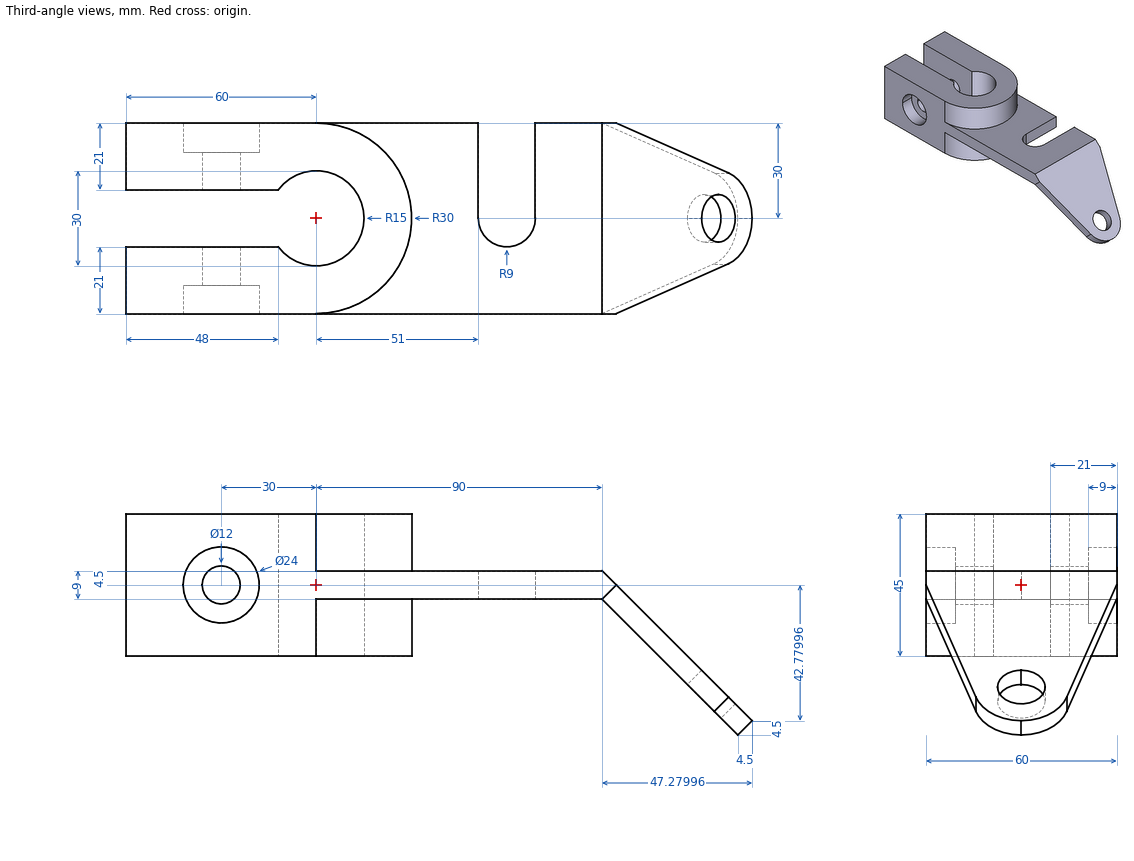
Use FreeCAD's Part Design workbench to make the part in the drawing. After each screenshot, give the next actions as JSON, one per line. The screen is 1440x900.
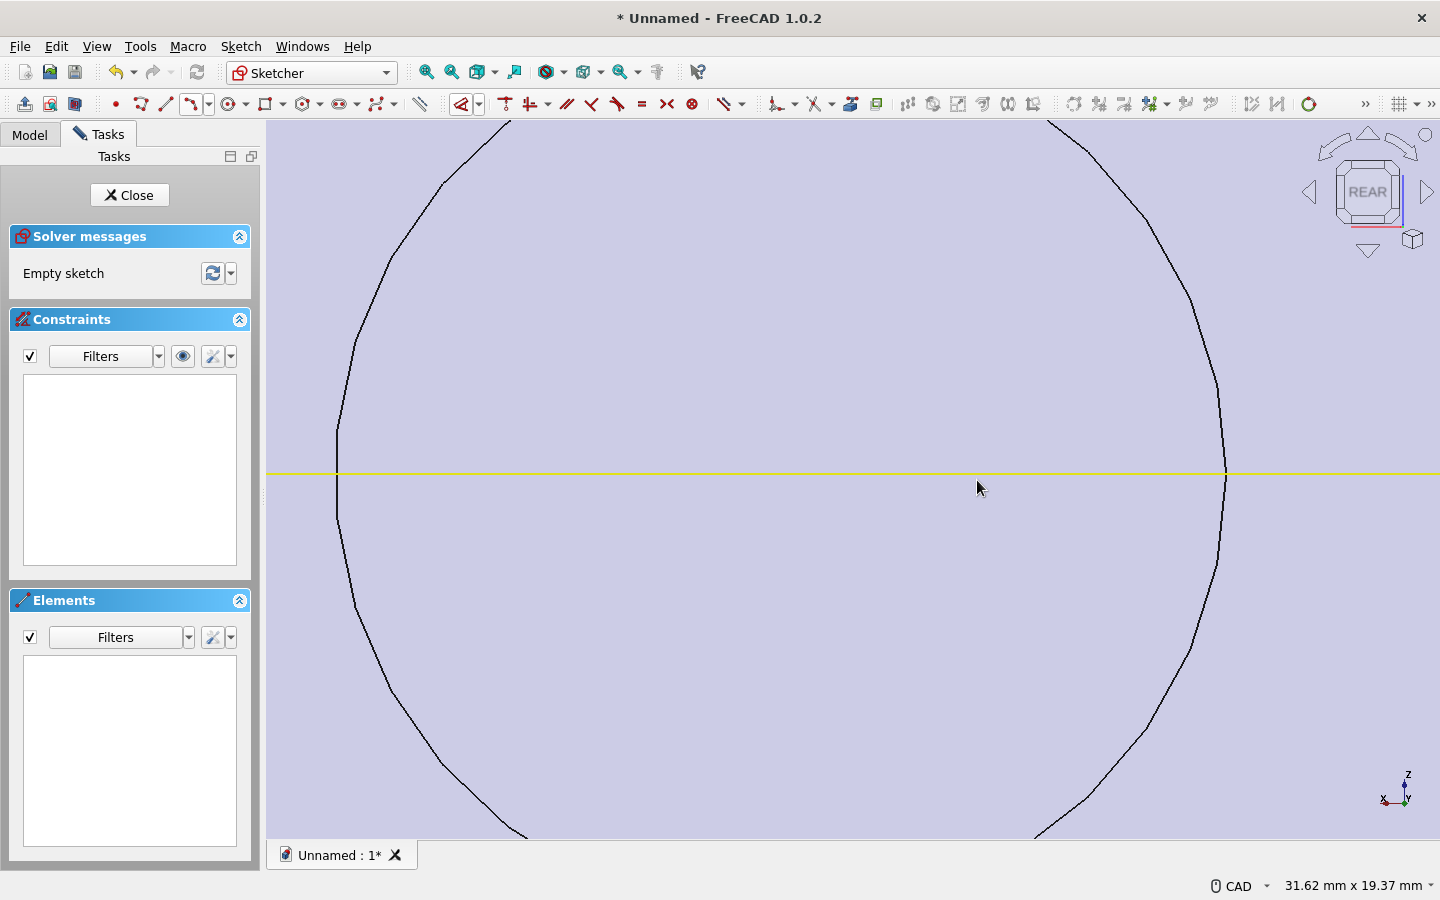
{"action": "key", "text": "g c"}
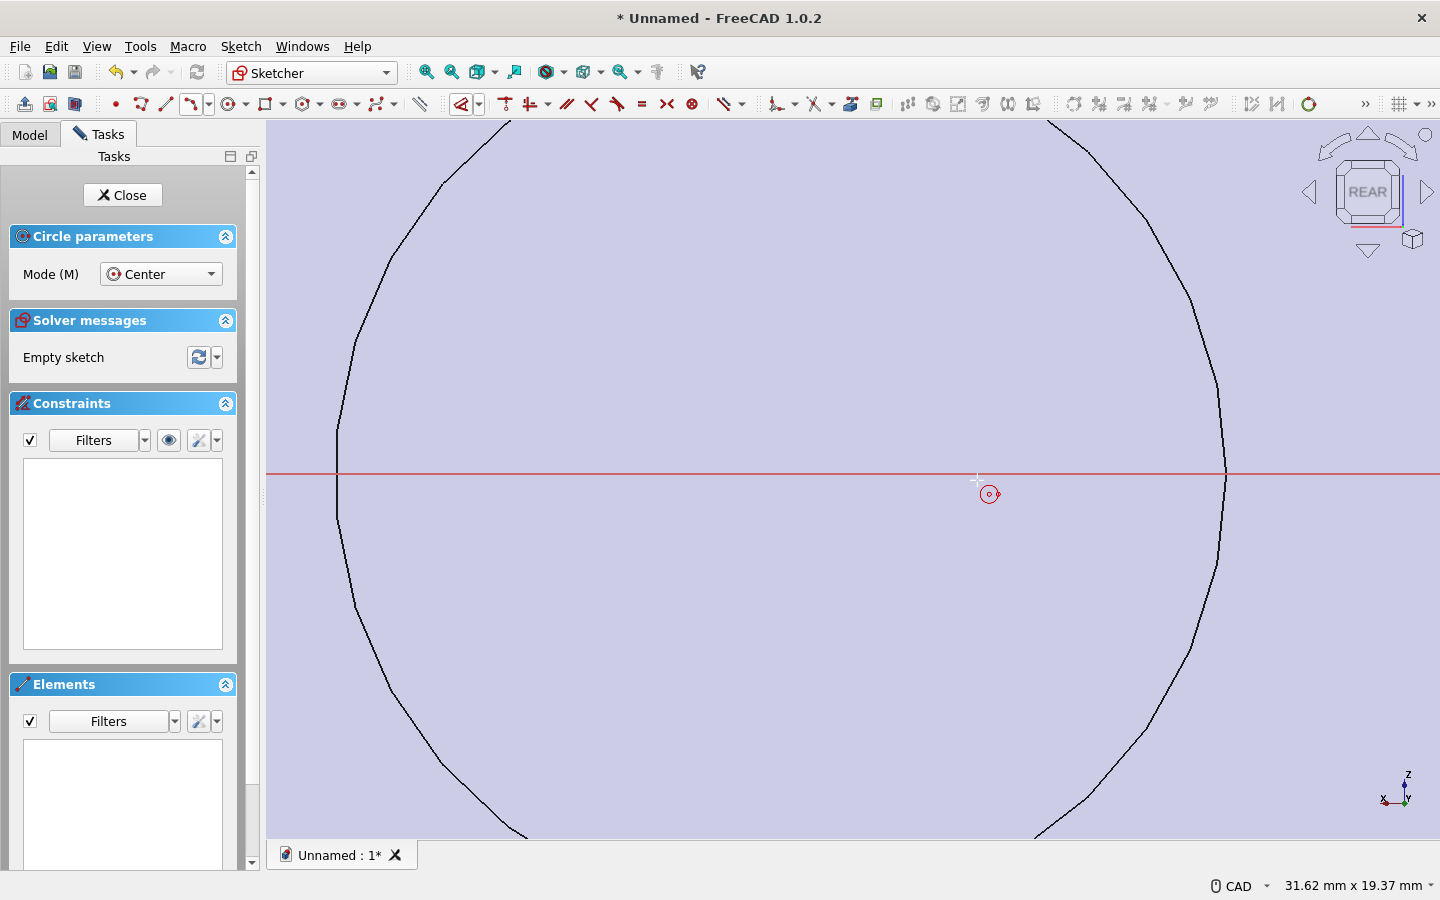
{"action": "left_click", "coordinate": [781, 474]}
{"action": "left_click", "coordinate": [938, 317]}
{"action": "key", "text": "Escape"}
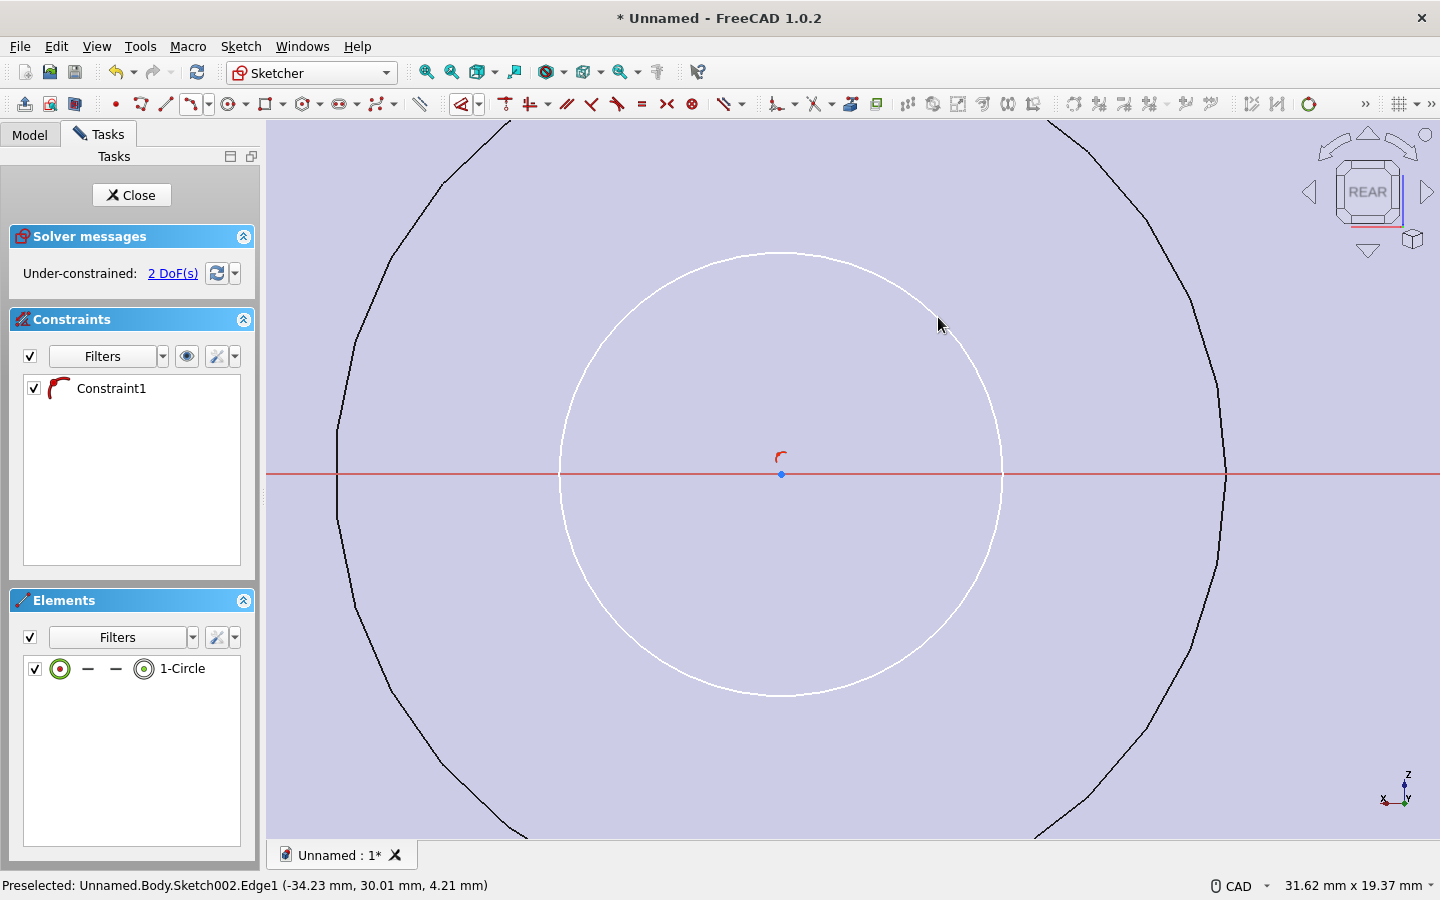
{"action": "left_click", "coordinate": [937, 317]}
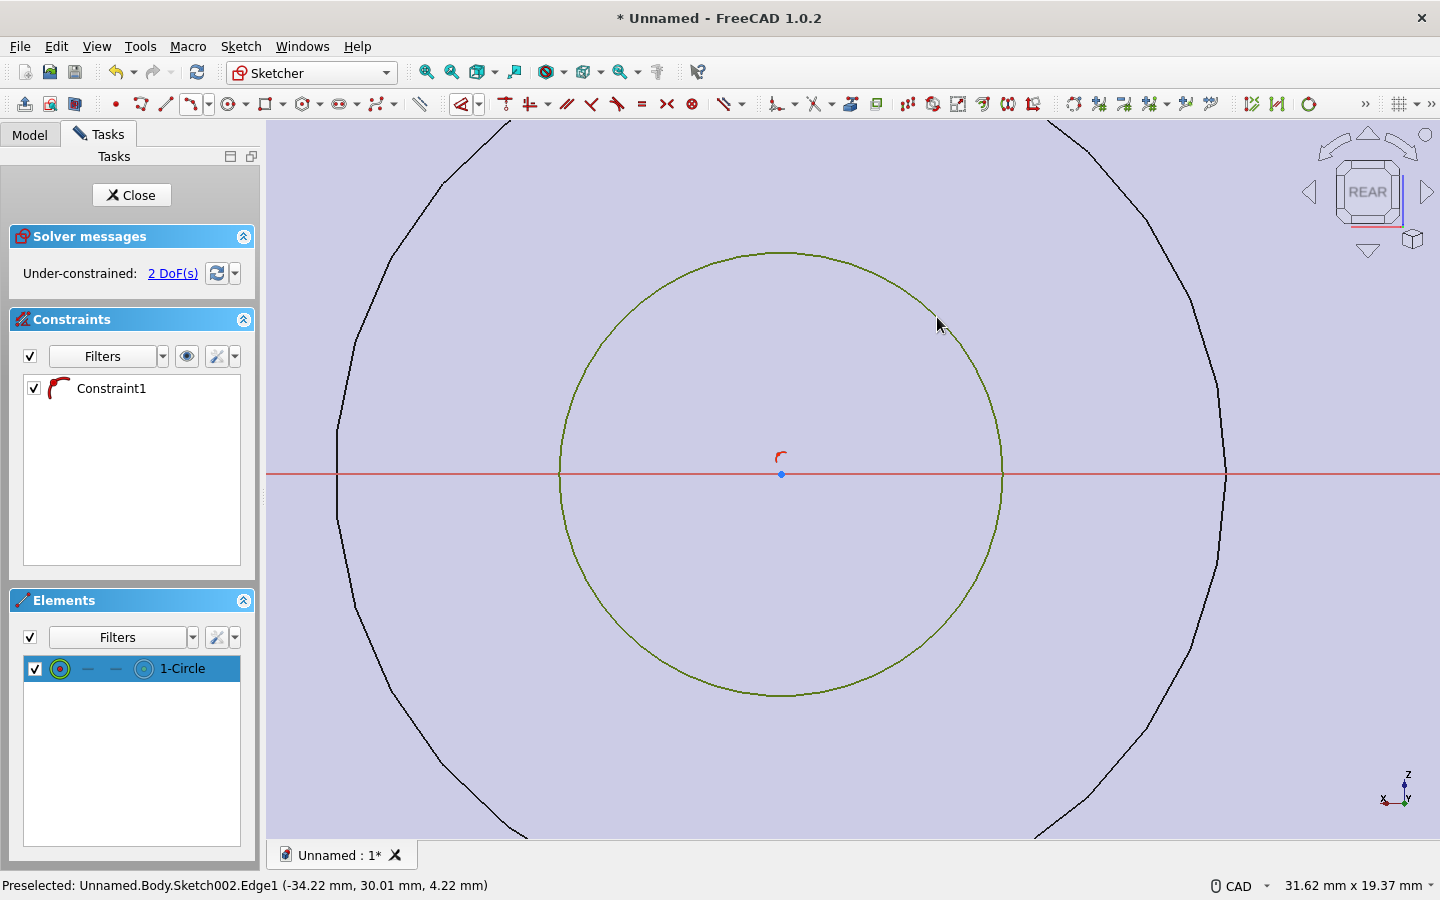
{"action": "left_click", "coordinate": [478, 104]}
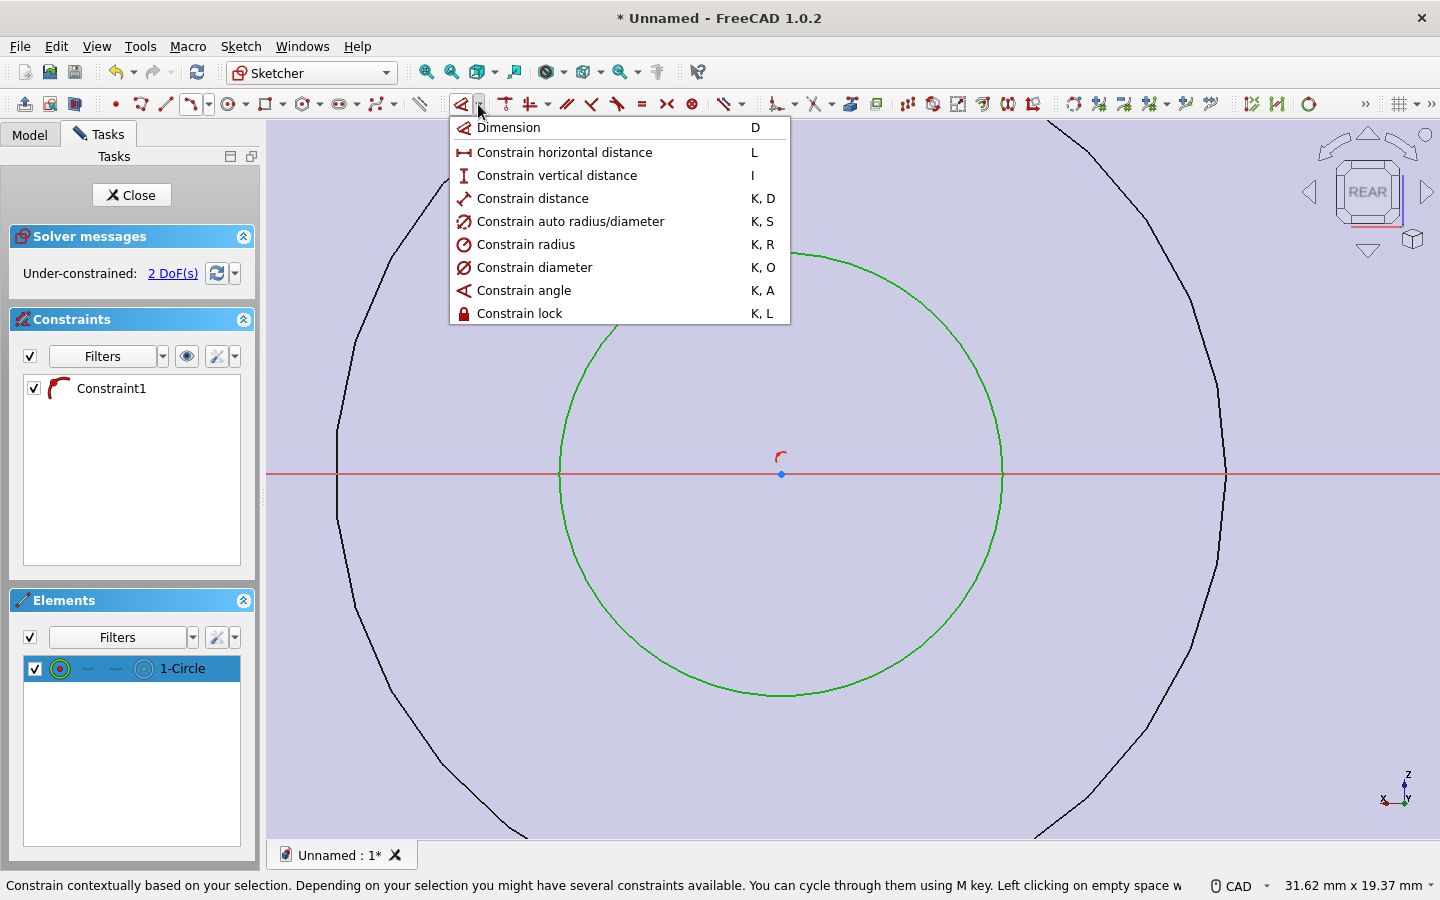
{"action": "left_click", "coordinate": [620, 268]}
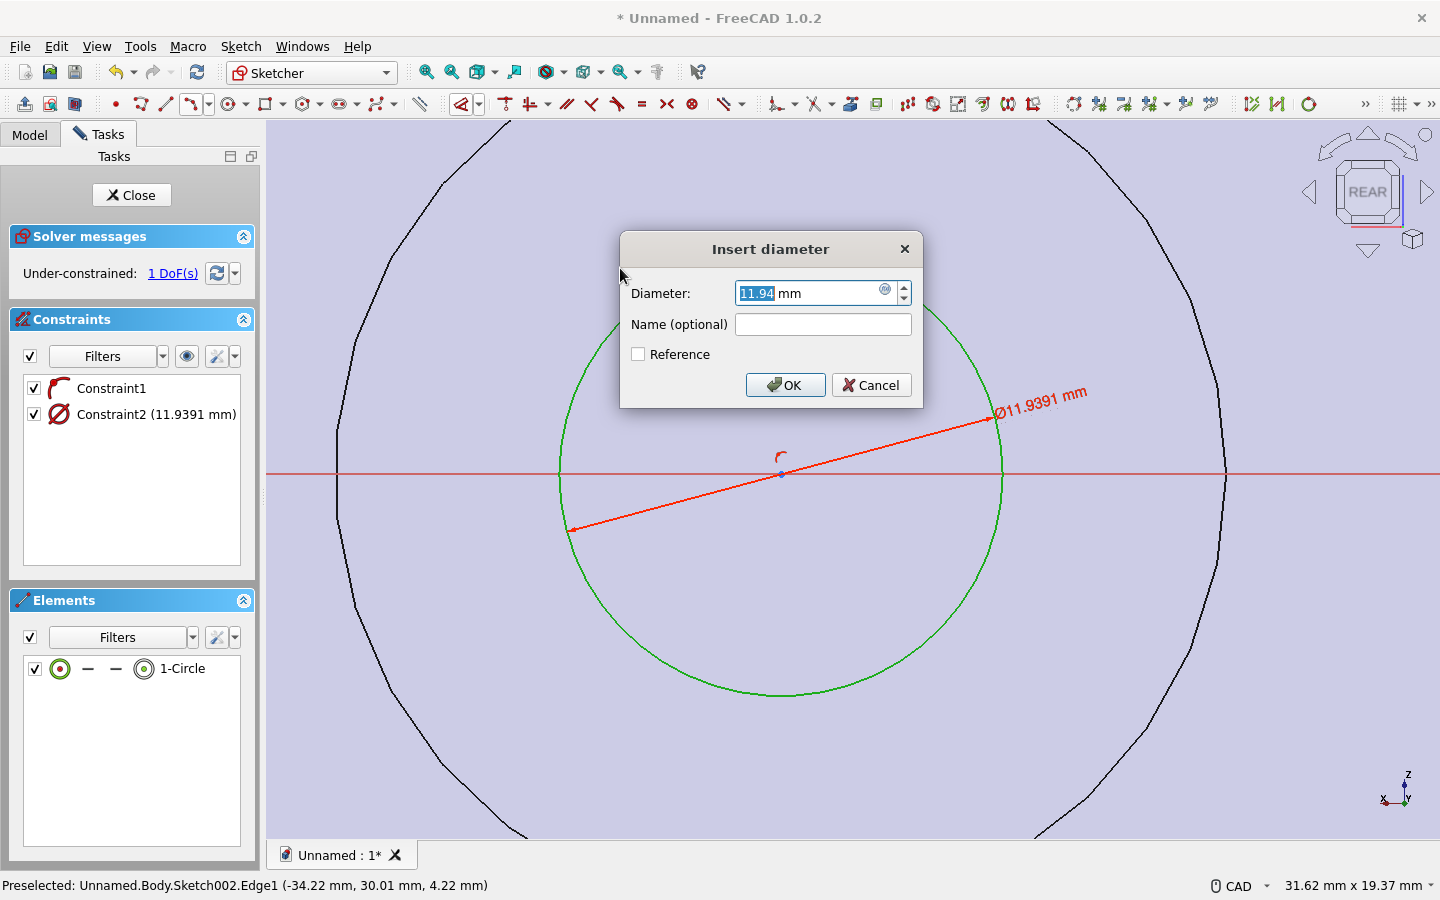
{"action": "type", "text": "12"}
{"action": "key", "text": "Return"}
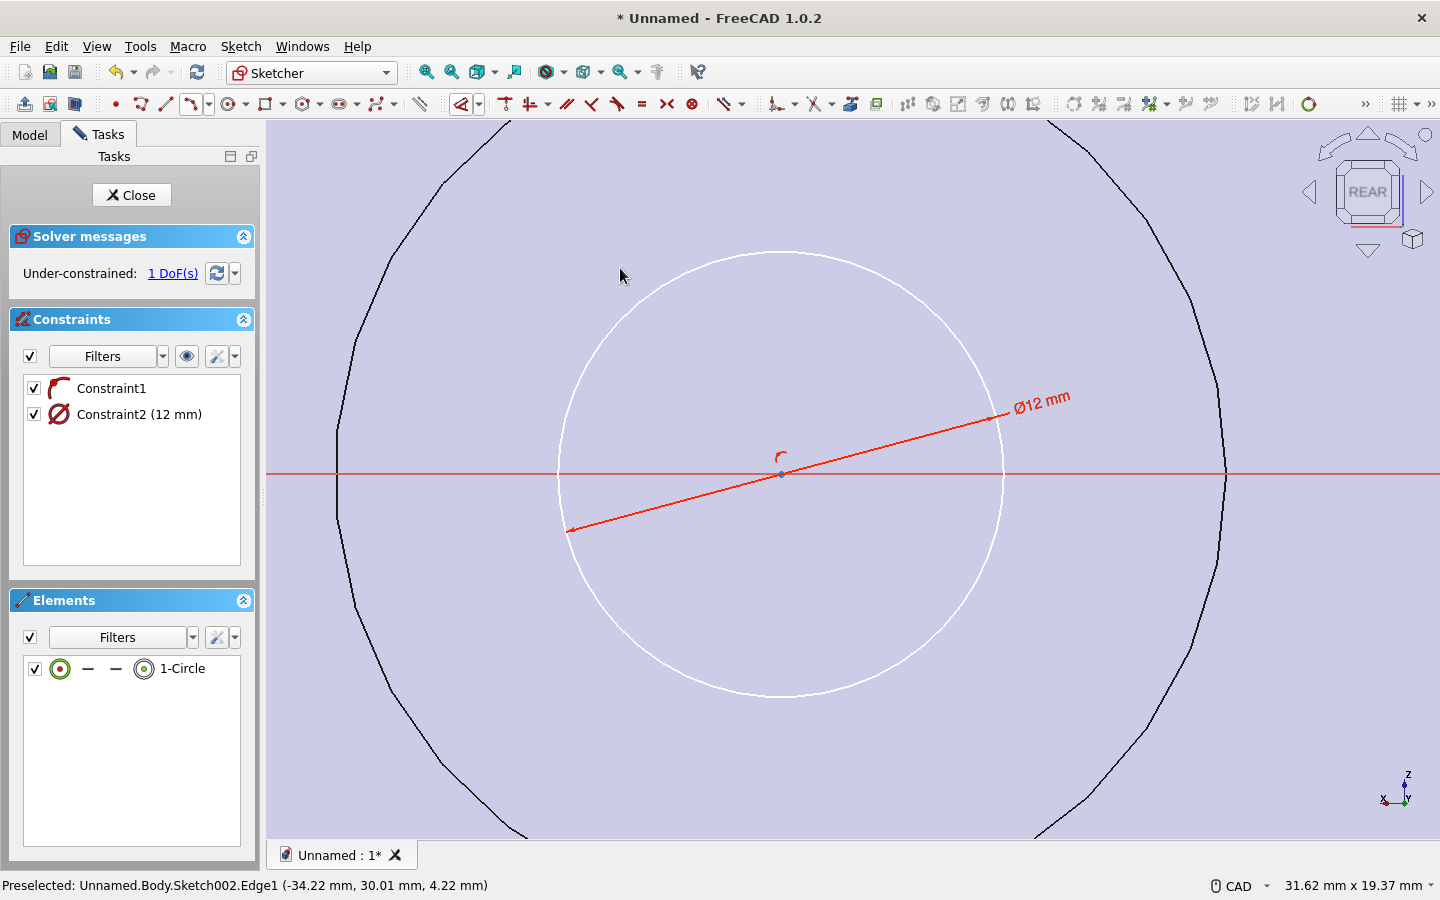
{"action": "left_click", "coordinate": [781, 474]}